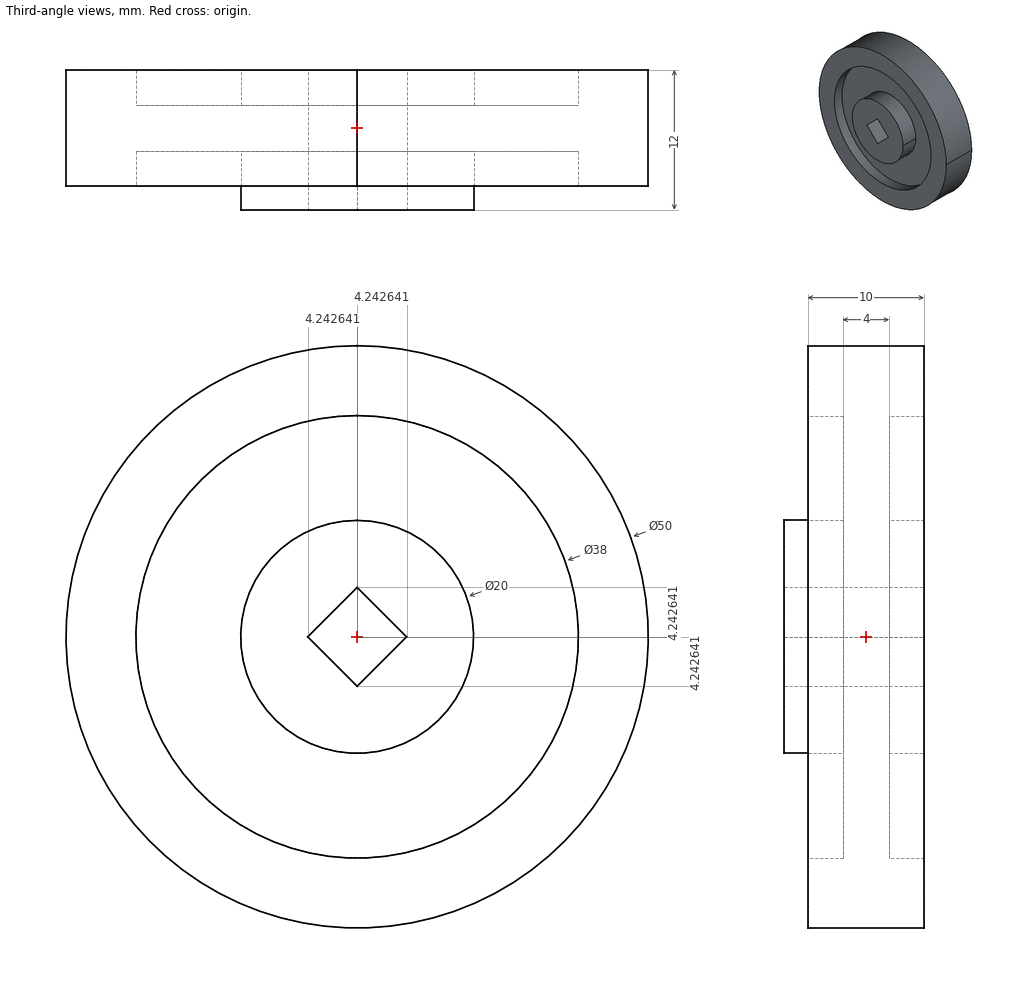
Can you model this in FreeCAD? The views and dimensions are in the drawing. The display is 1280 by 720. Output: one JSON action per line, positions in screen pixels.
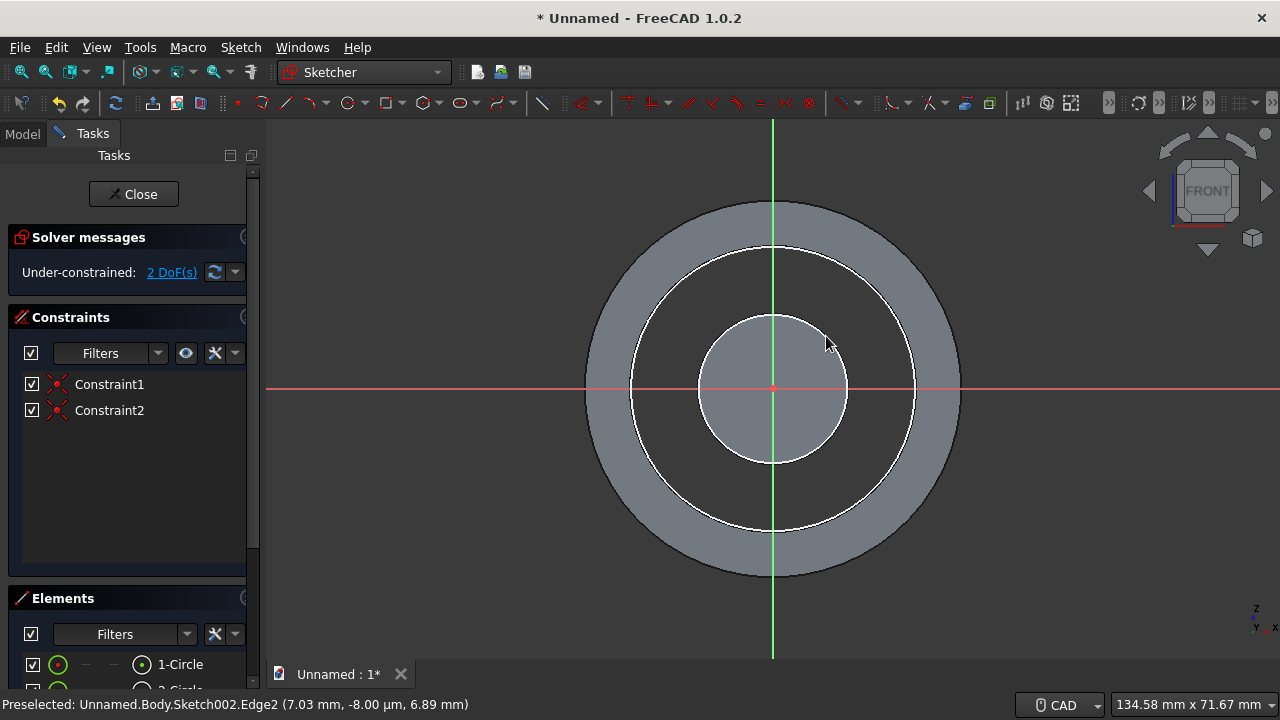
{"action": "key", "text": "d"}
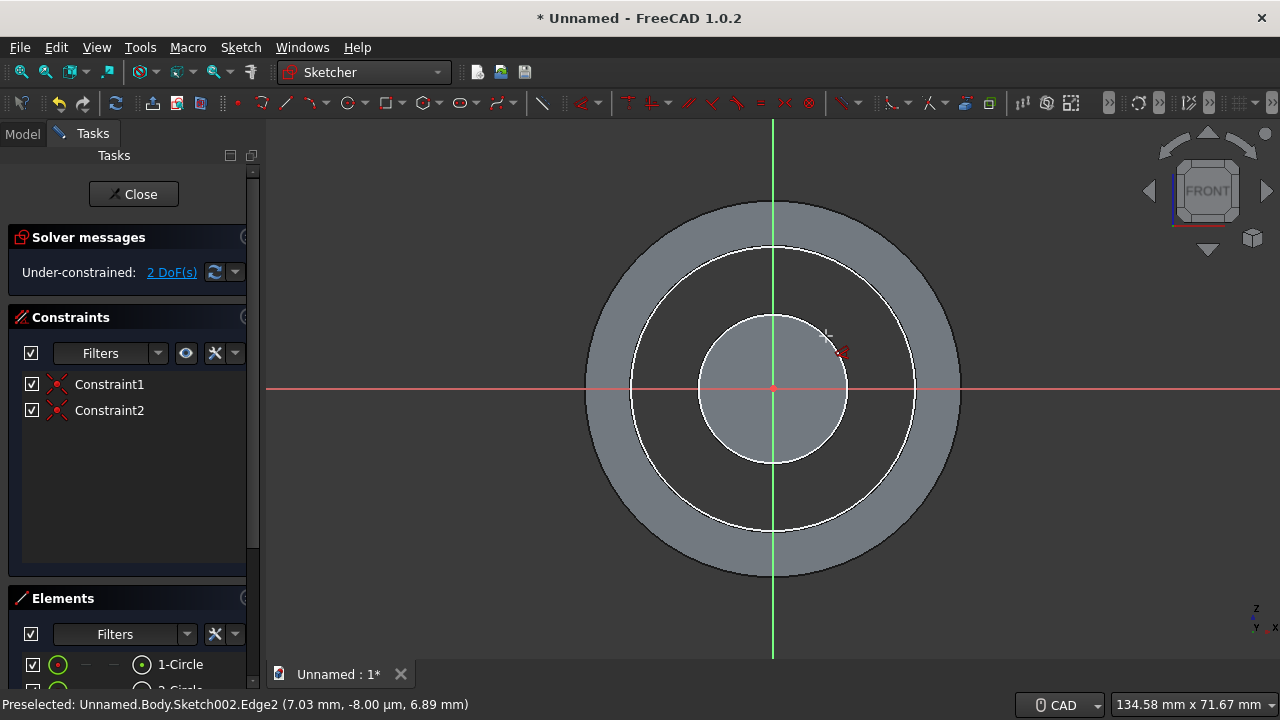
{"action": "left_click", "coordinate": [873, 288]}
{"action": "left_click", "coordinate": [896, 265]}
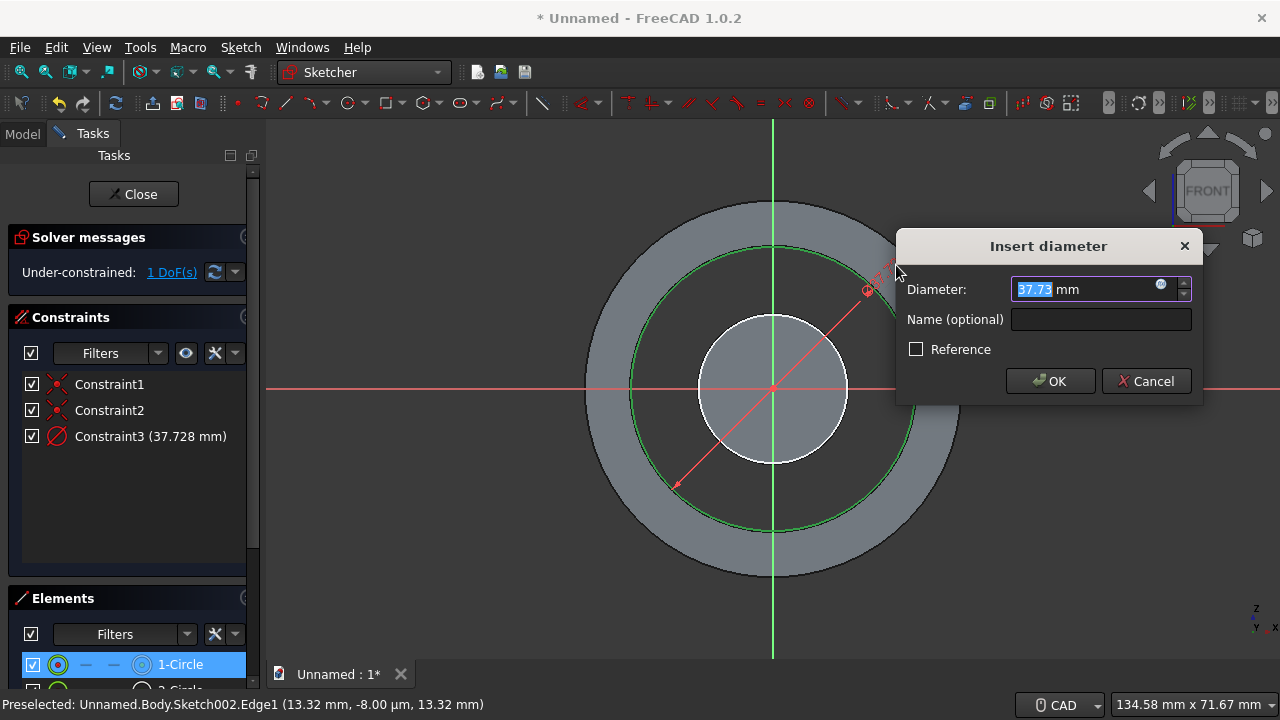
{"action": "type", "text": "38"}
{"action": "key", "text": "Return"}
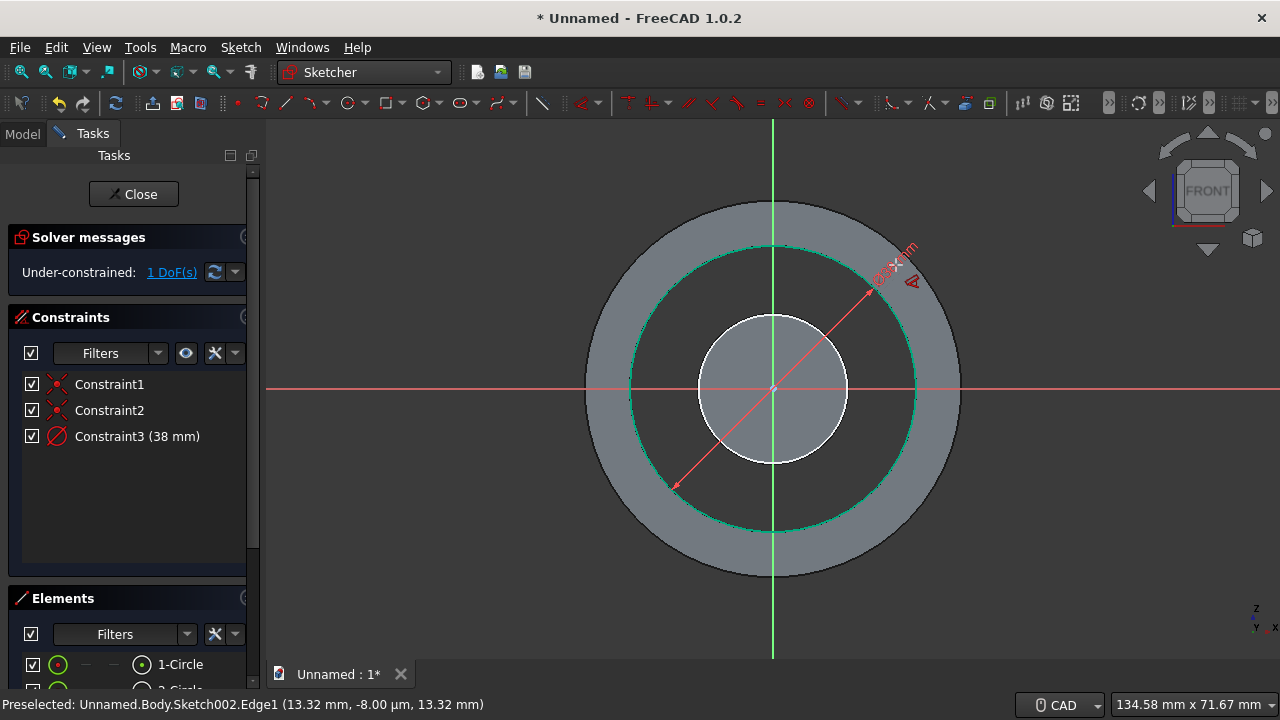
{"action": "left_click", "coordinate": [825, 336]}
{"action": "left_click", "coordinate": [847, 313]}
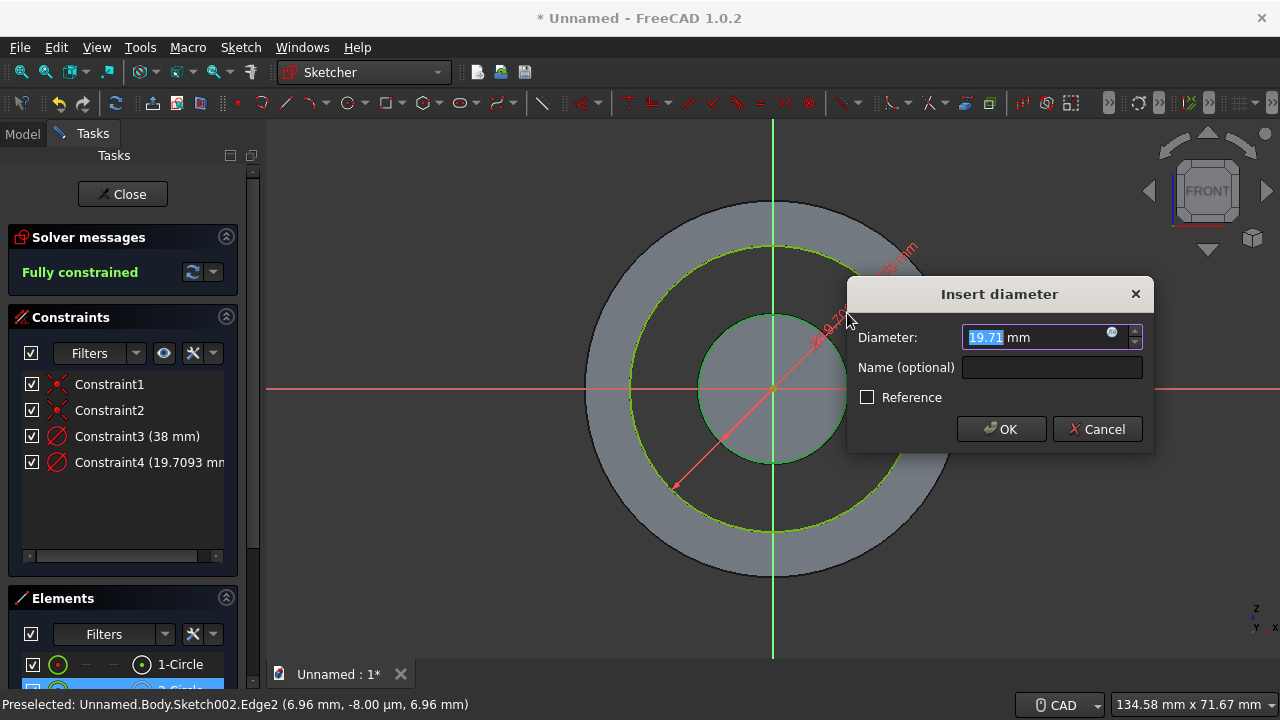
{"action": "type", "text": "20"}
{"action": "key", "text": "Return"}
{"action": "key", "text": "Escape"}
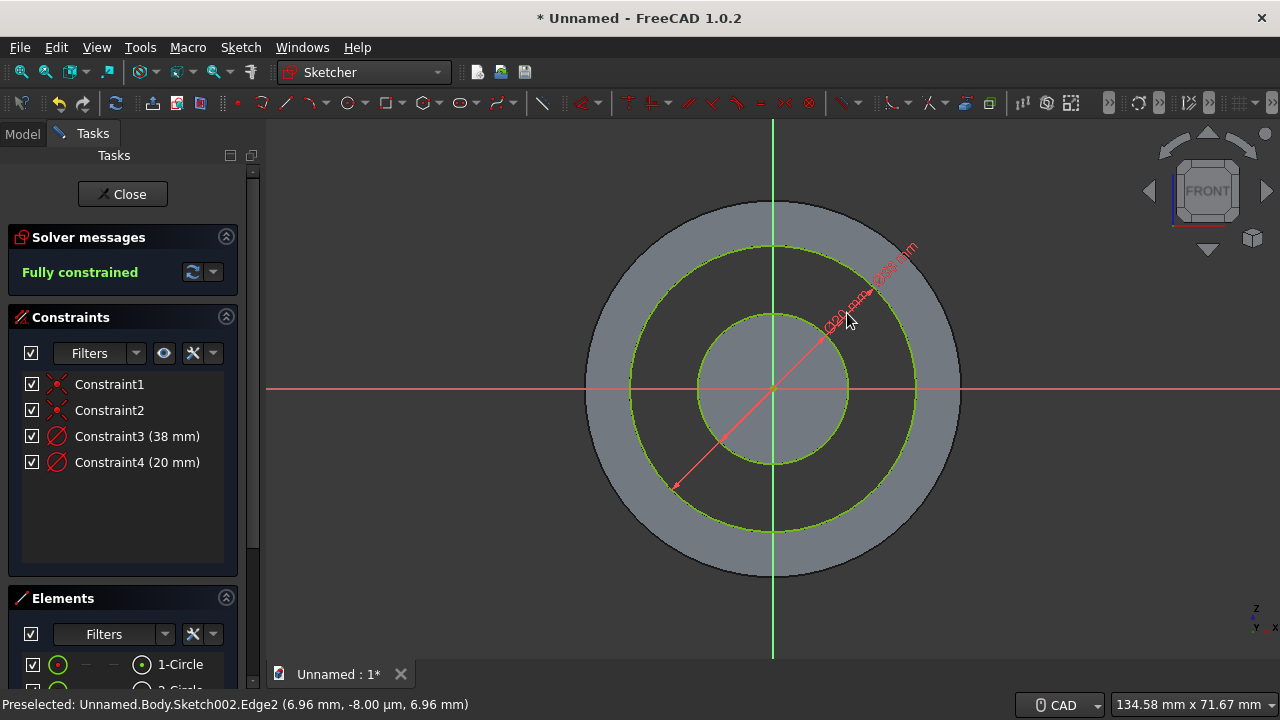
{"action": "left_click", "coordinate": [123, 194]}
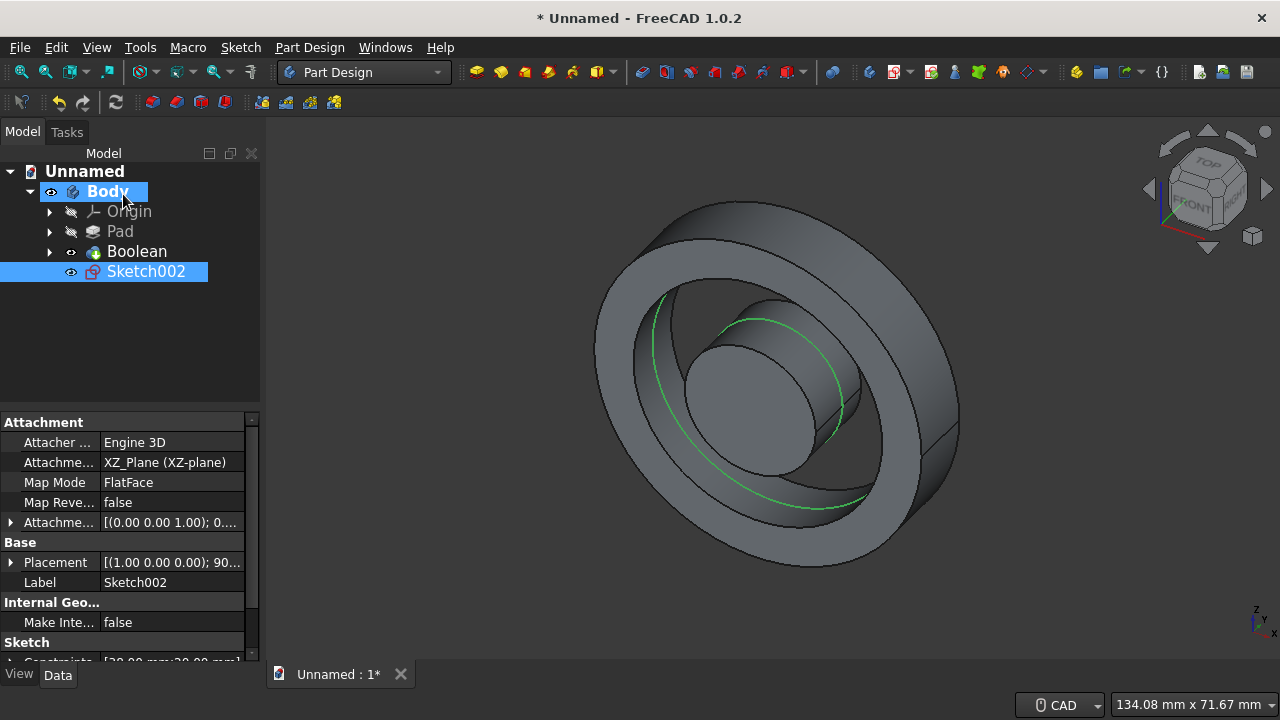
{"action": "left_click", "coordinate": [478, 72]}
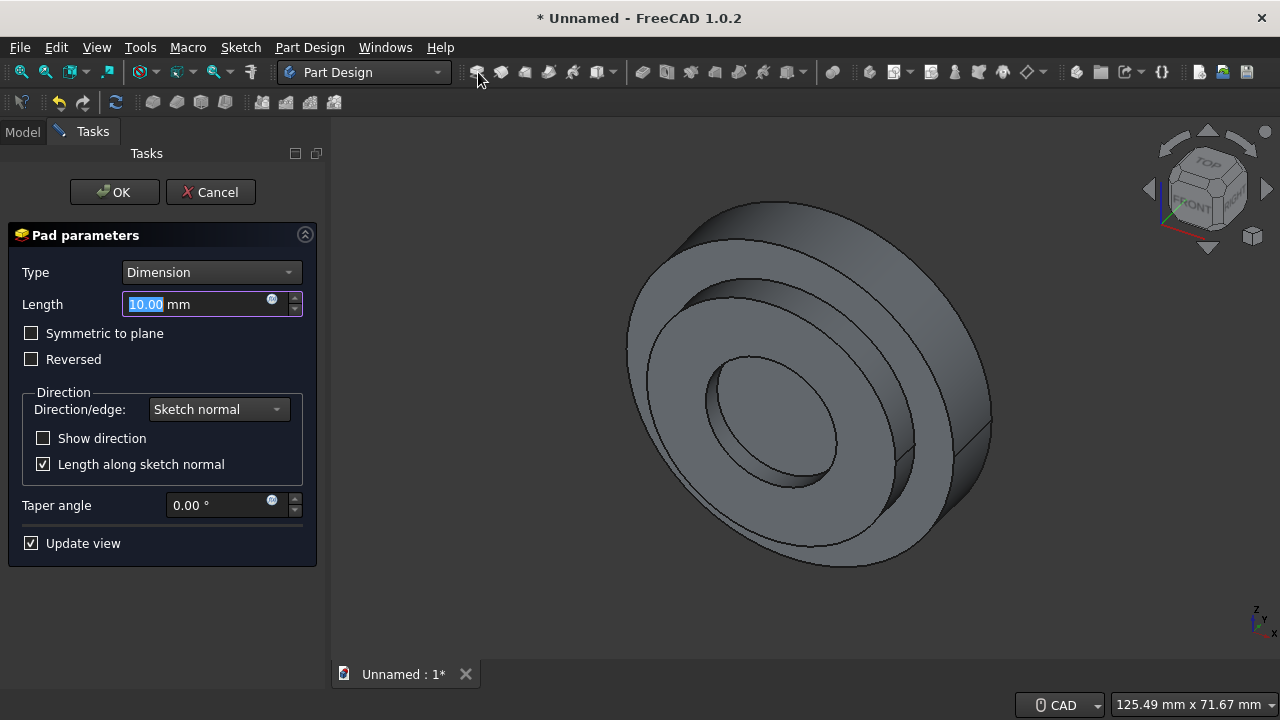
{"action": "type", "text": "4"}
{"action": "key", "text": "Tab"}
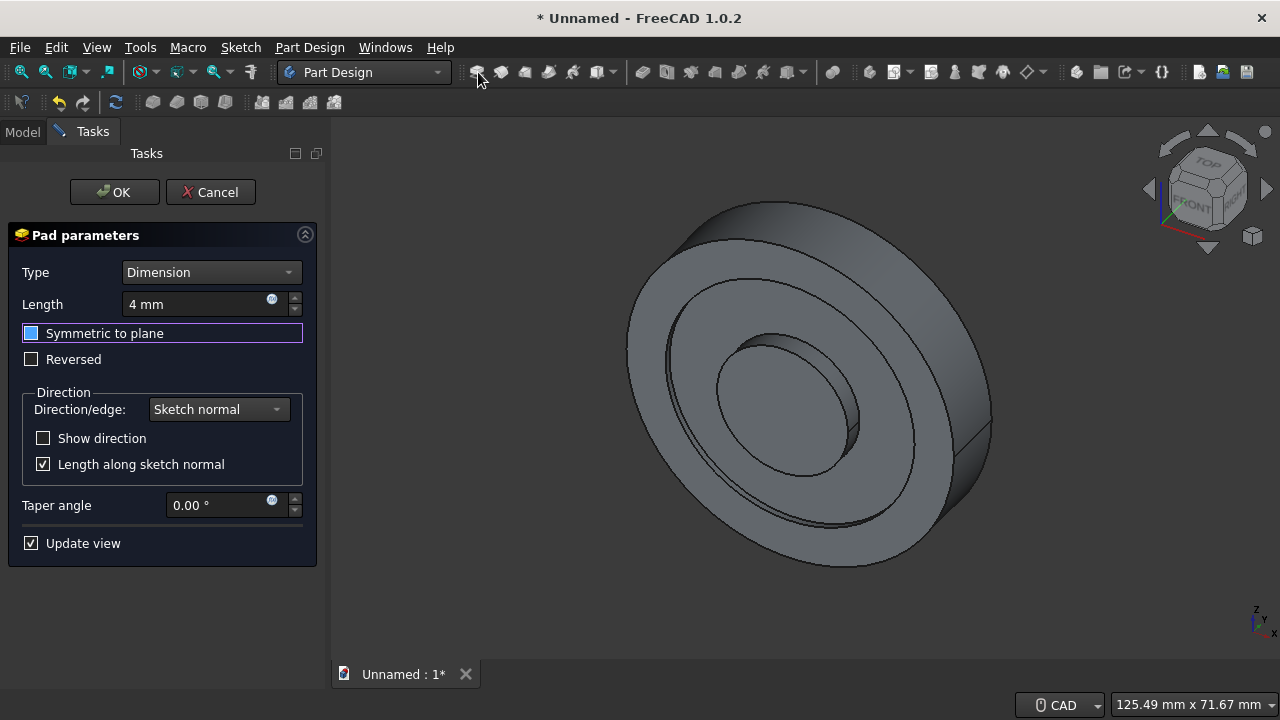
{"action": "left_click", "coordinate": [30, 333]}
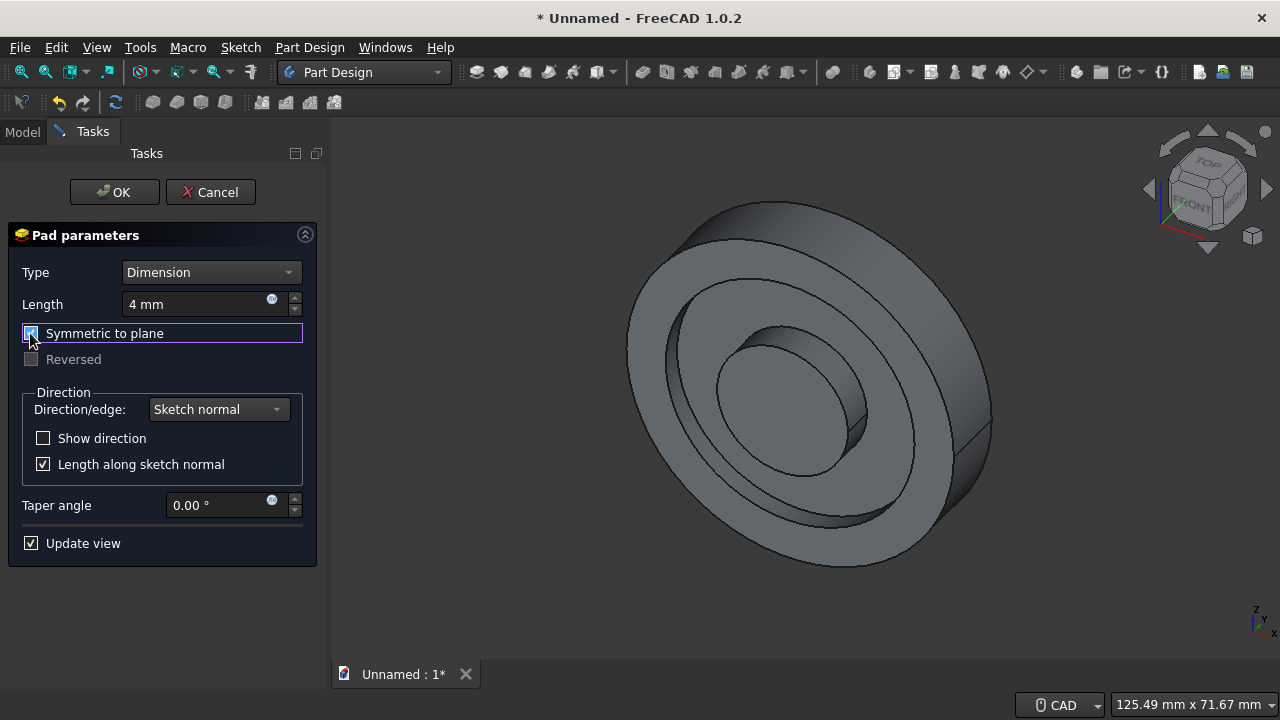
{"action": "left_click", "coordinate": [115, 192]}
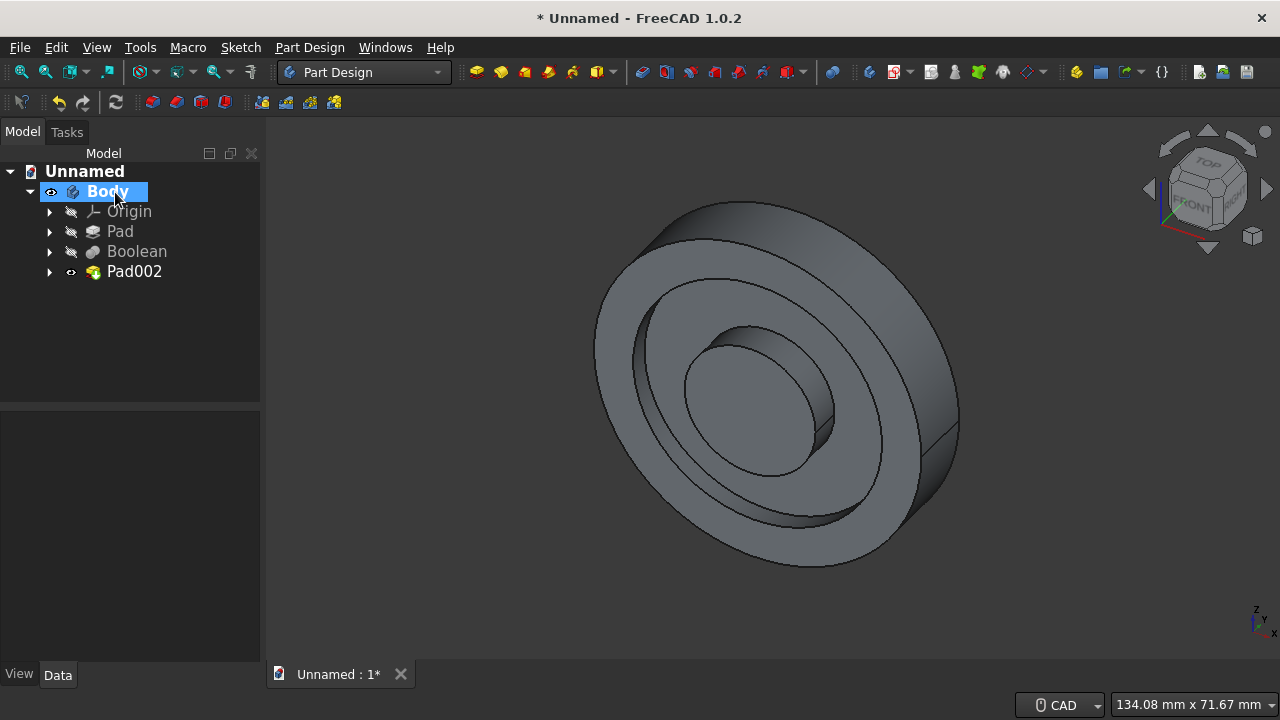
{"action": "left_click", "coordinate": [750, 410]}